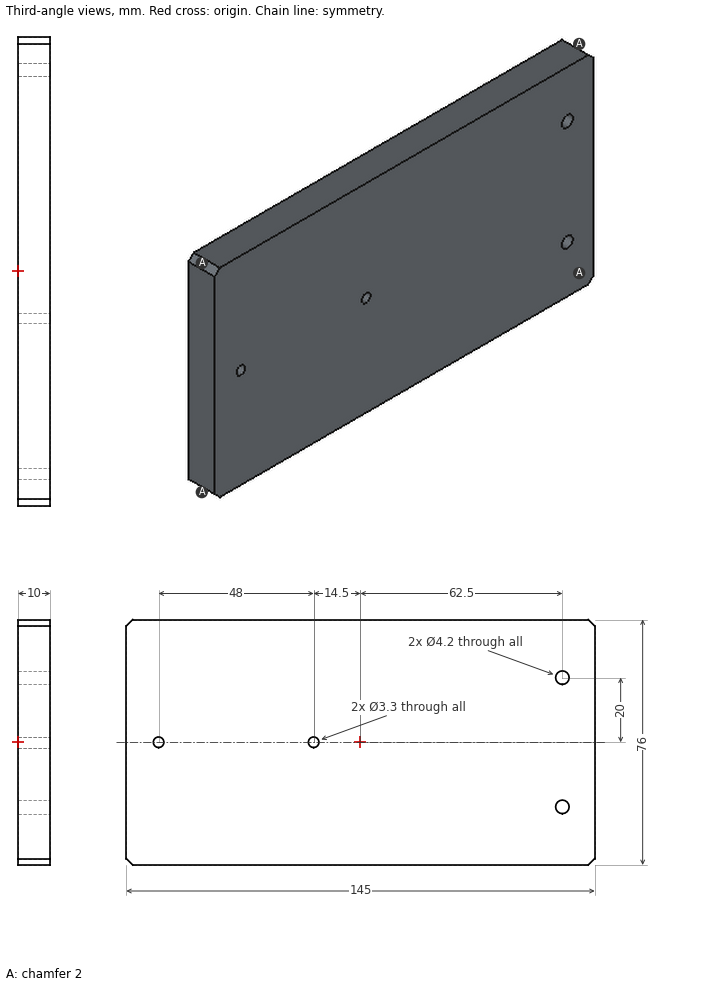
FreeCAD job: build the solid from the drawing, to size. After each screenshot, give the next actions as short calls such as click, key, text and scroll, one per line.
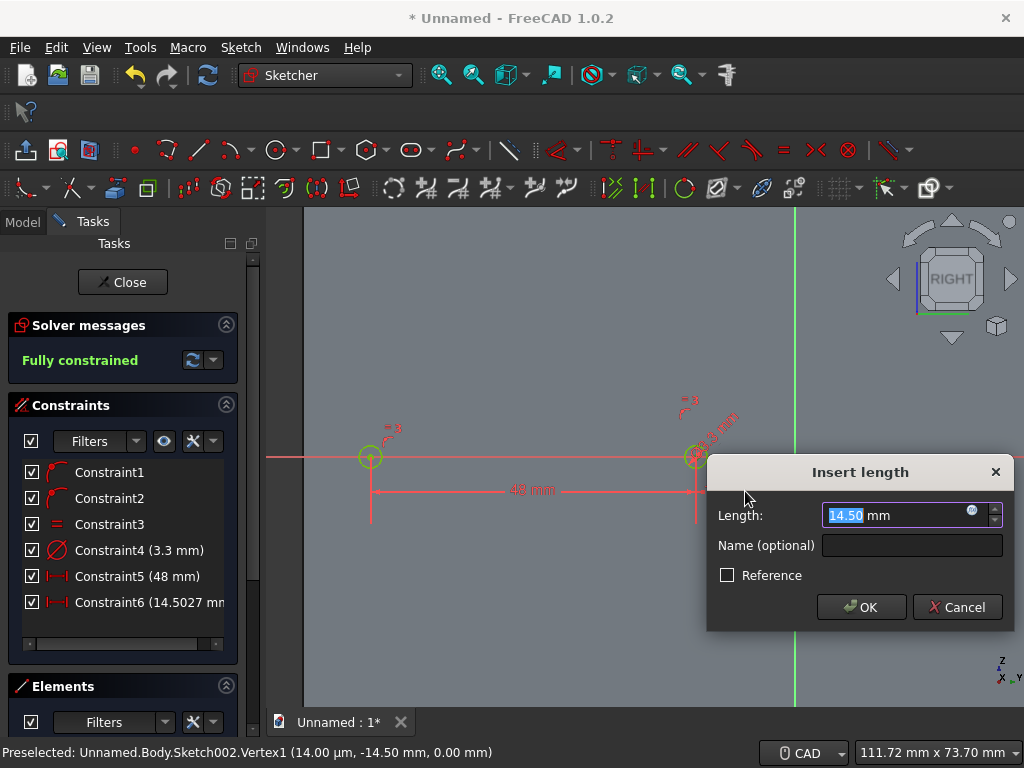
text(14.5)
key(Return)
key(Escape)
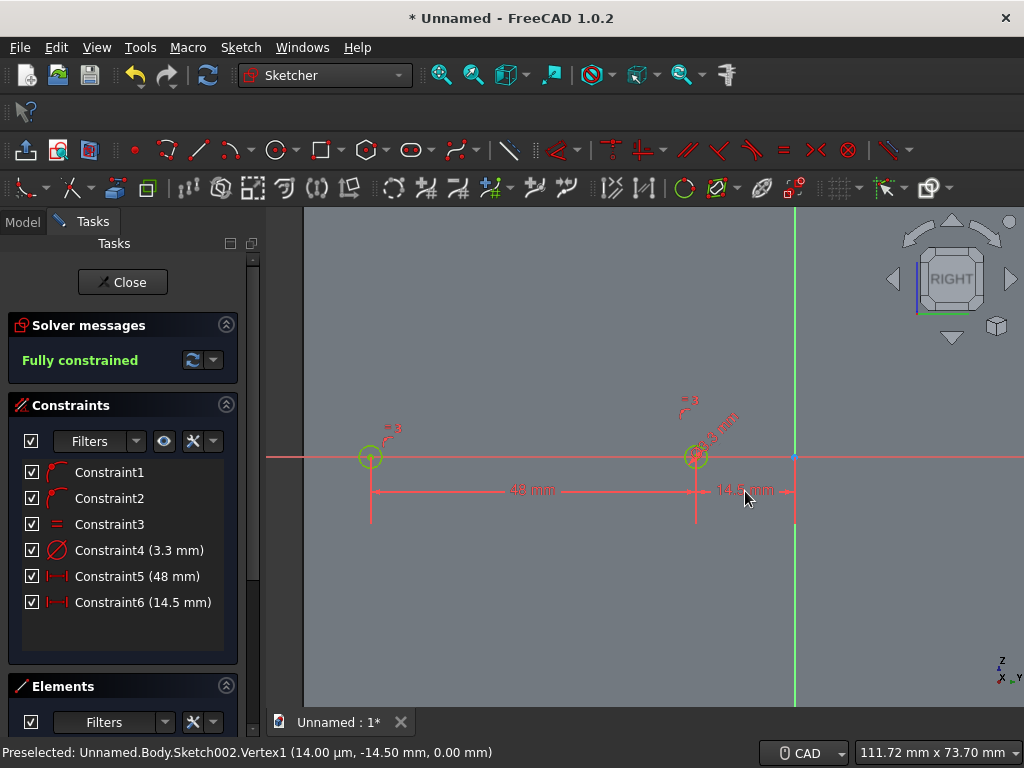
click(123, 282)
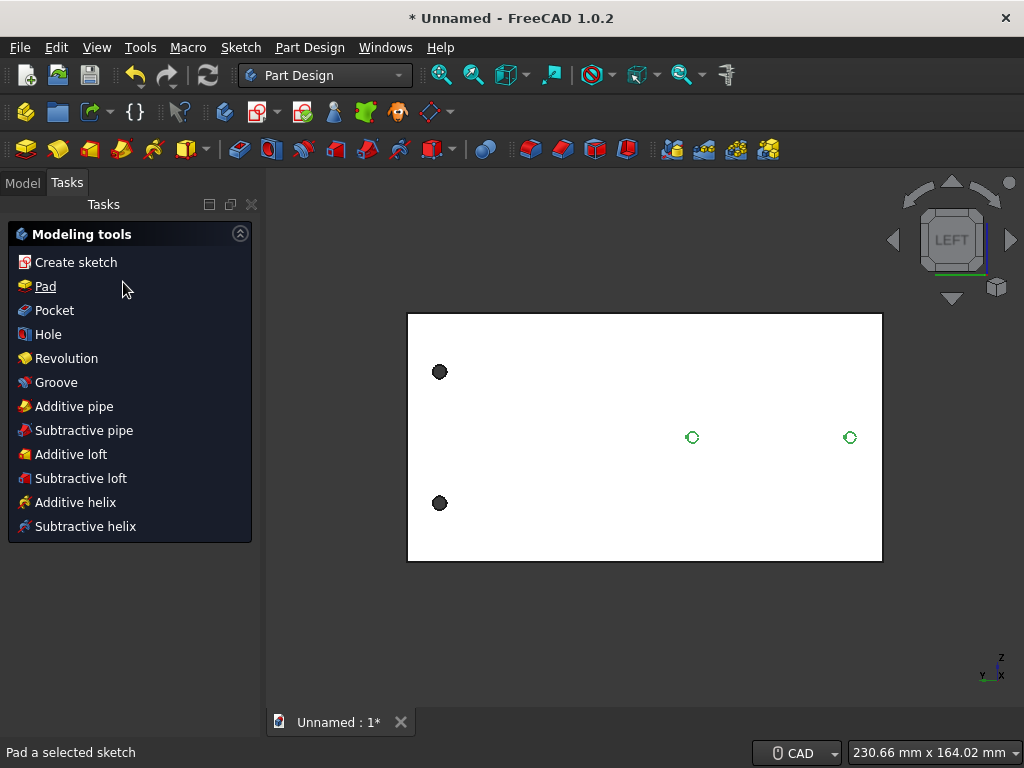
click(272, 150)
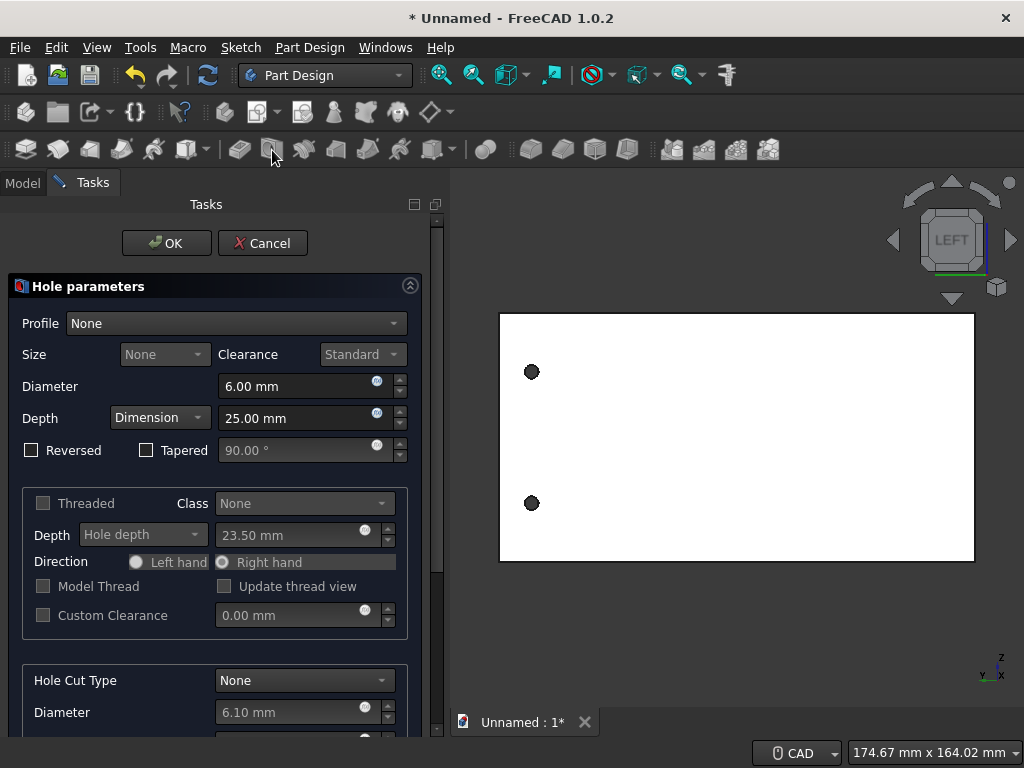
triple_click(305, 386)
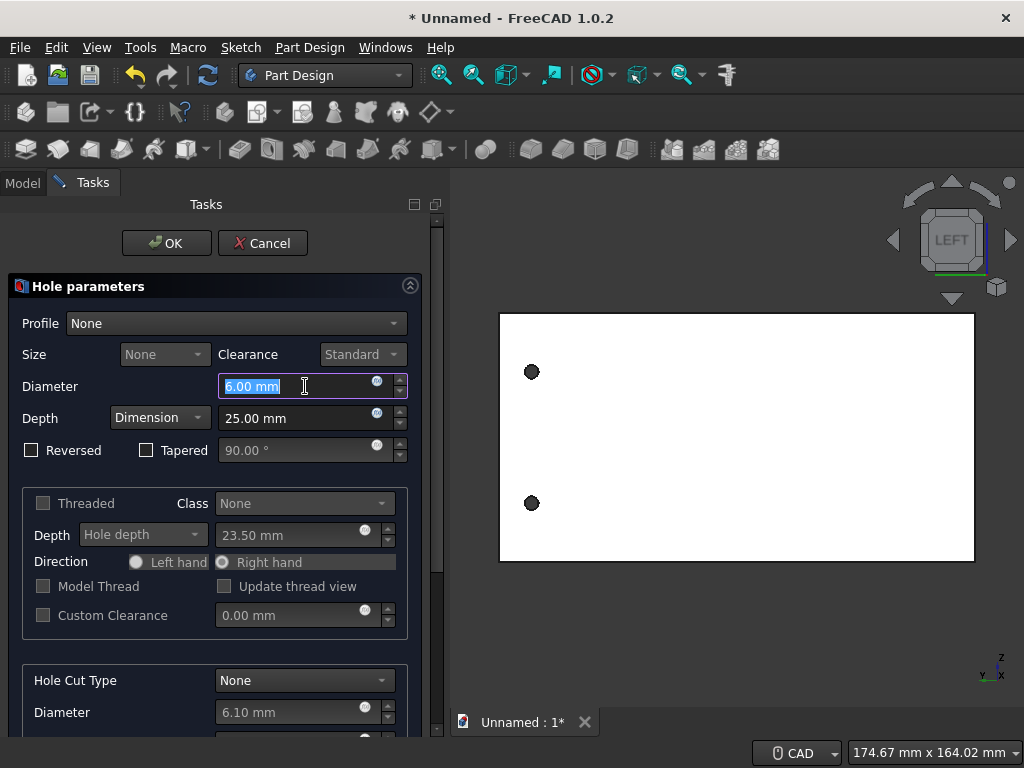
text(3.3)
key(Tab)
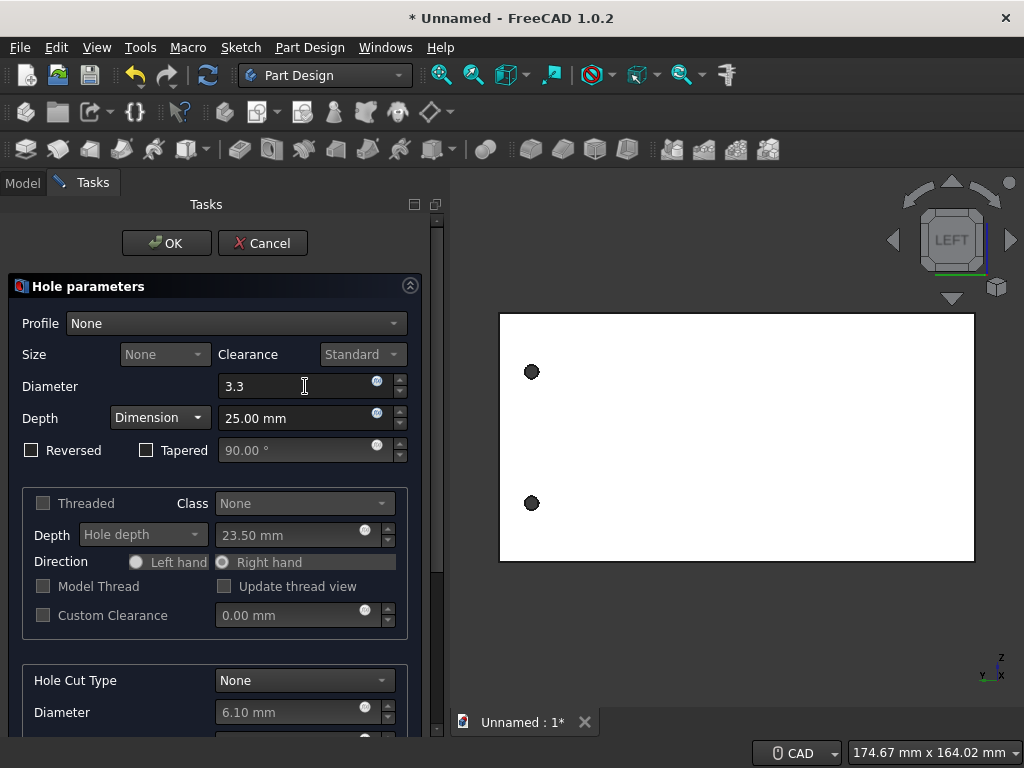
click(161, 418)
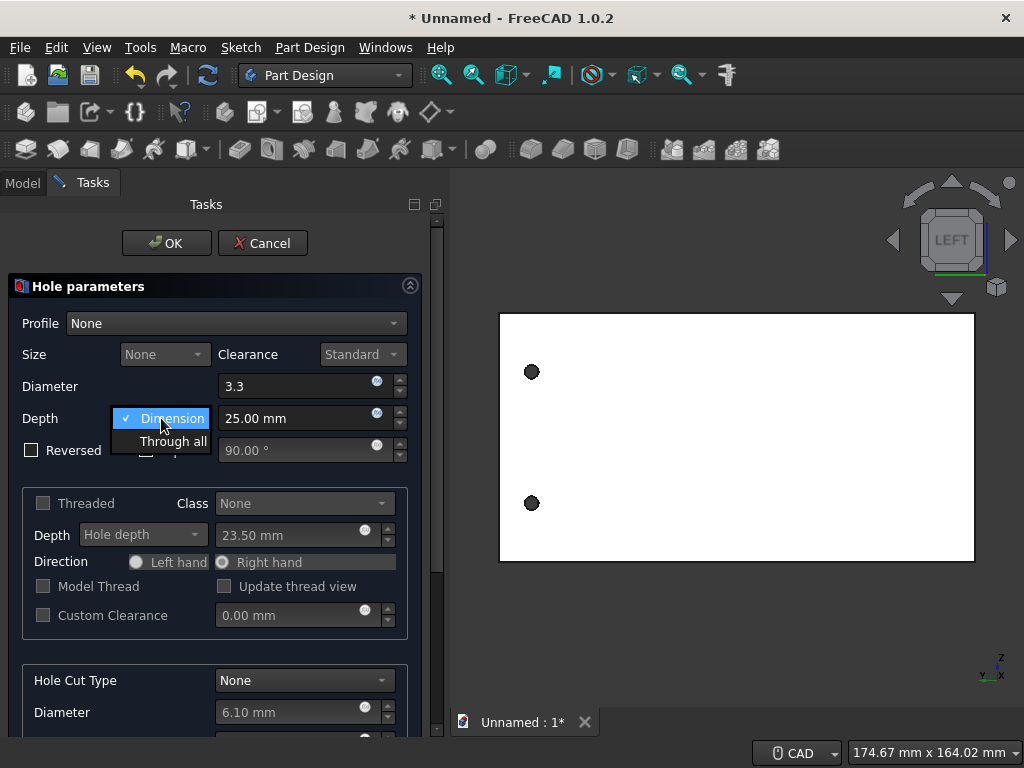
click(160, 442)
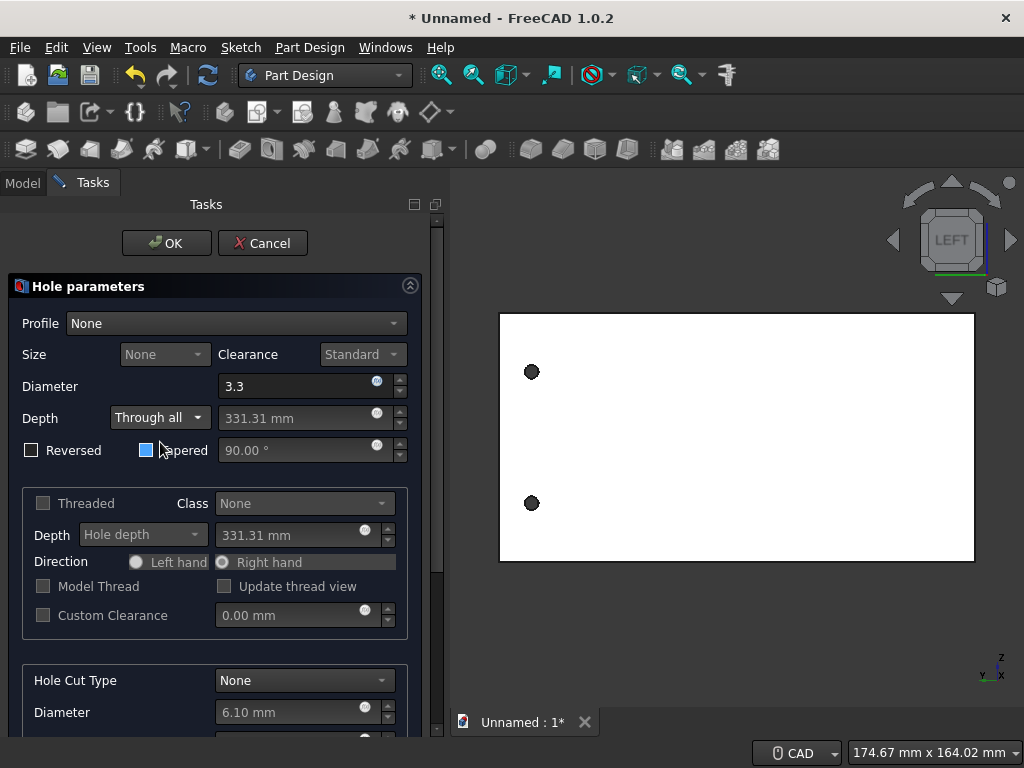
click(30, 450)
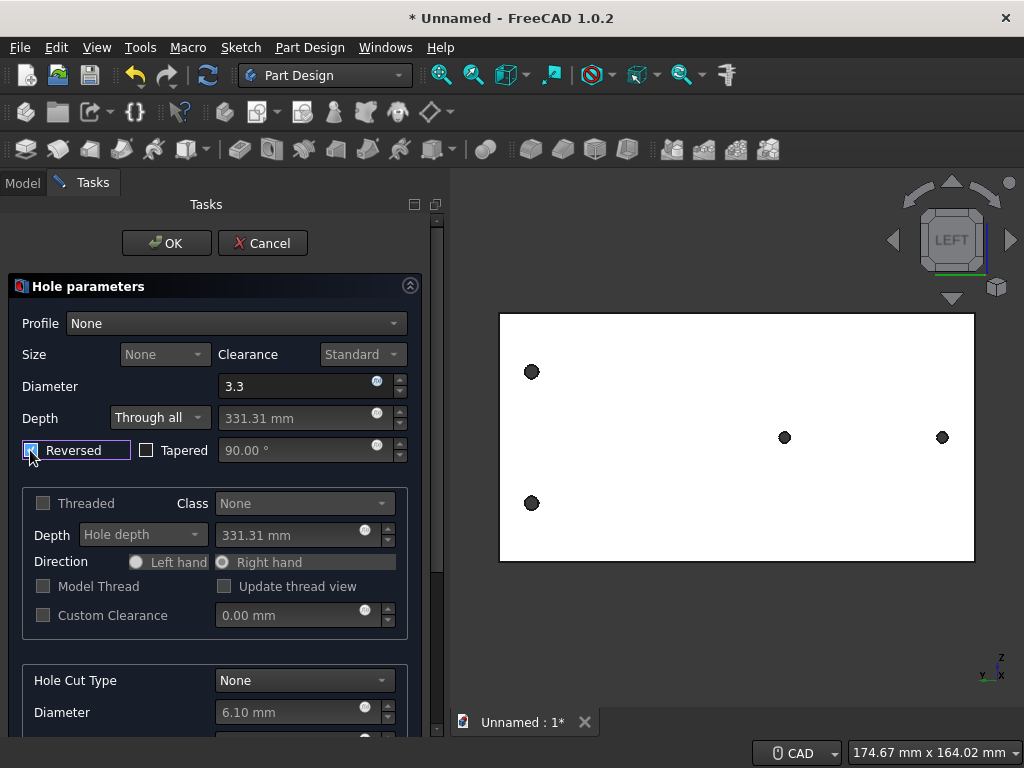
click(167, 243)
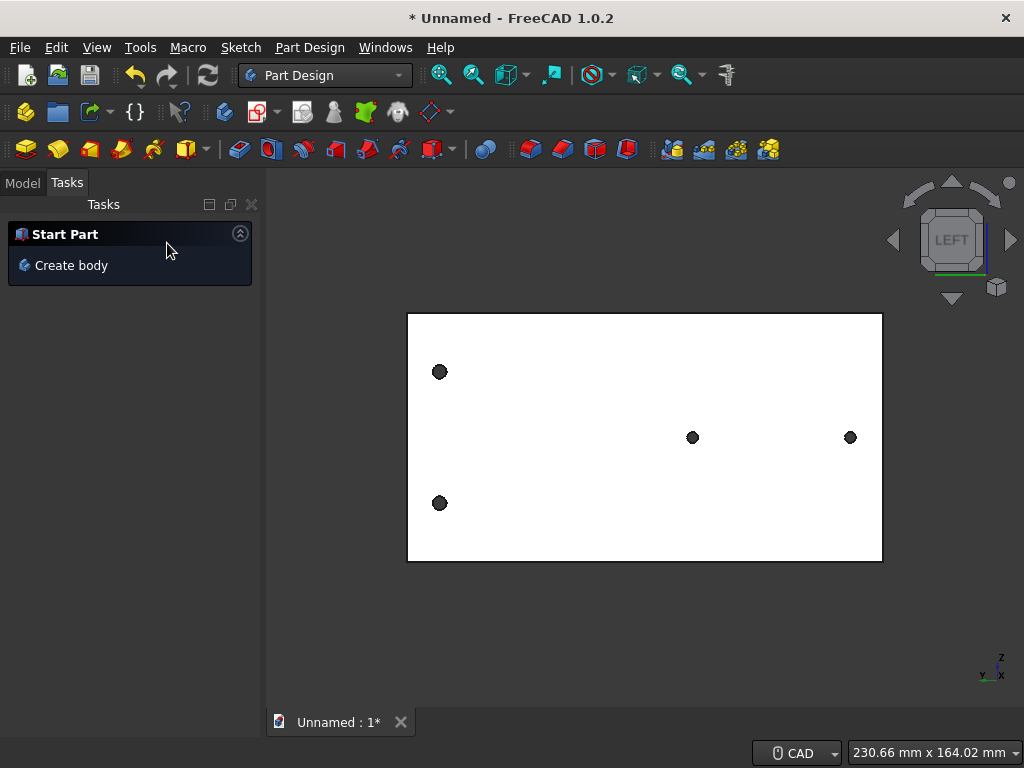
key(0)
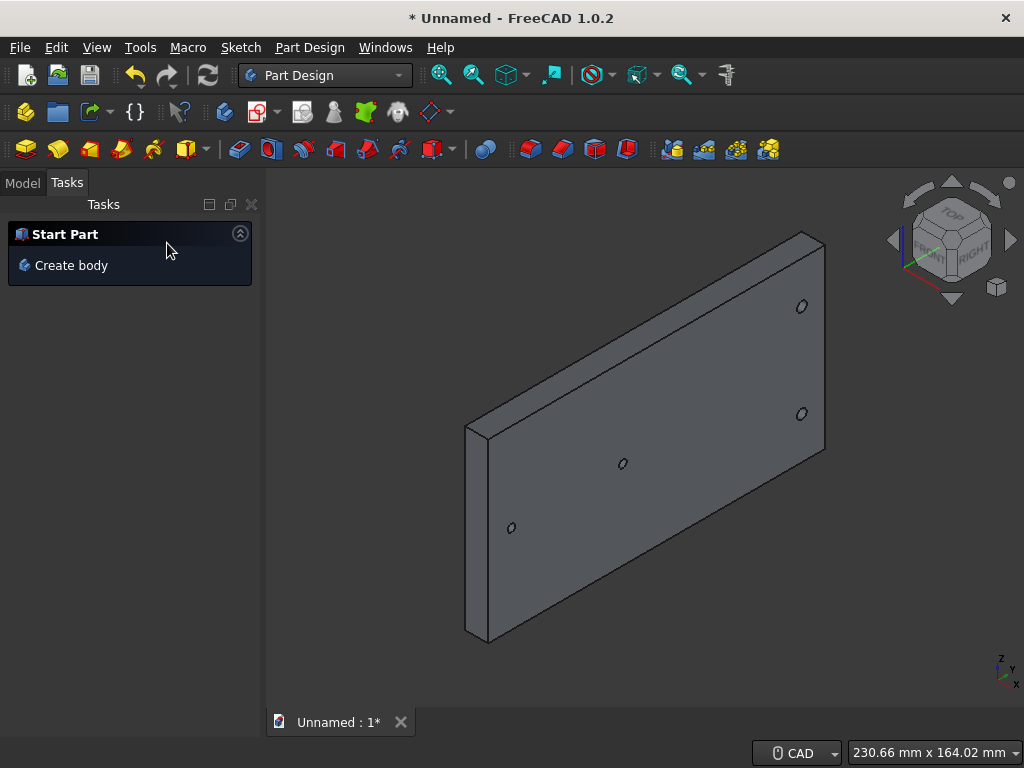
click(477, 432)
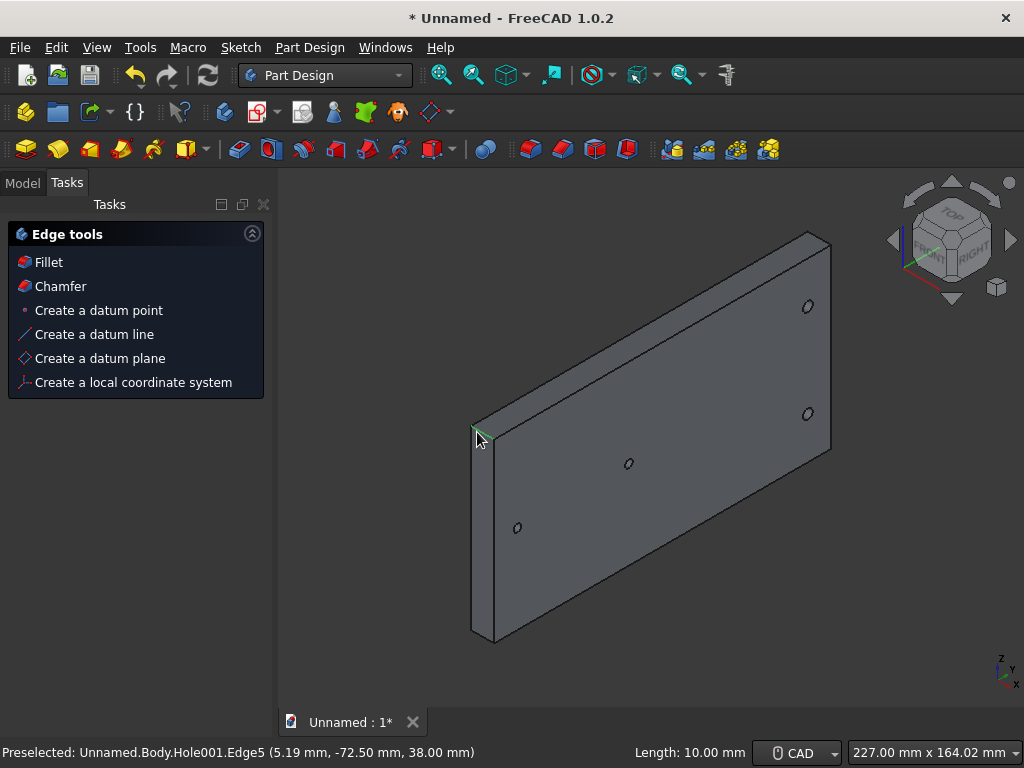
key(2)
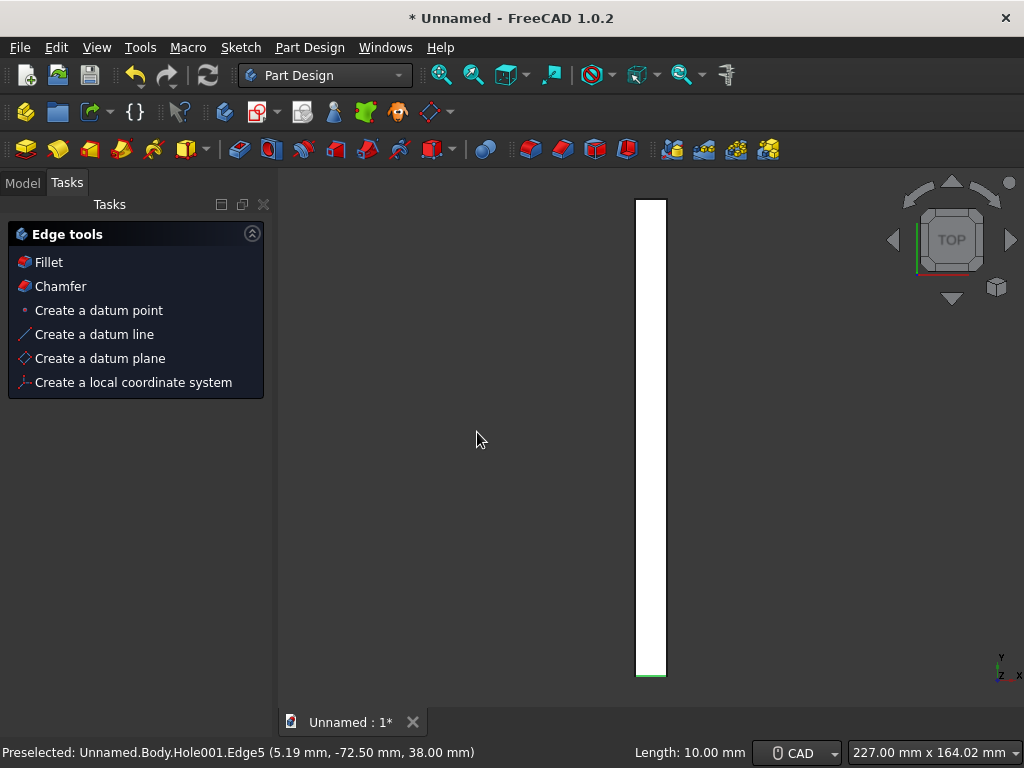
click(651, 198, ctrl)